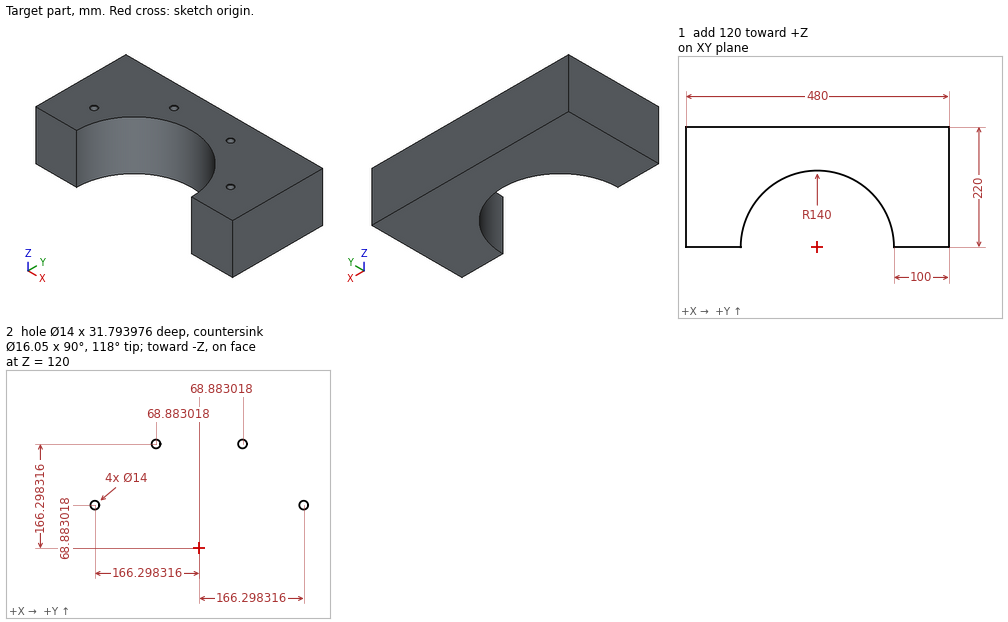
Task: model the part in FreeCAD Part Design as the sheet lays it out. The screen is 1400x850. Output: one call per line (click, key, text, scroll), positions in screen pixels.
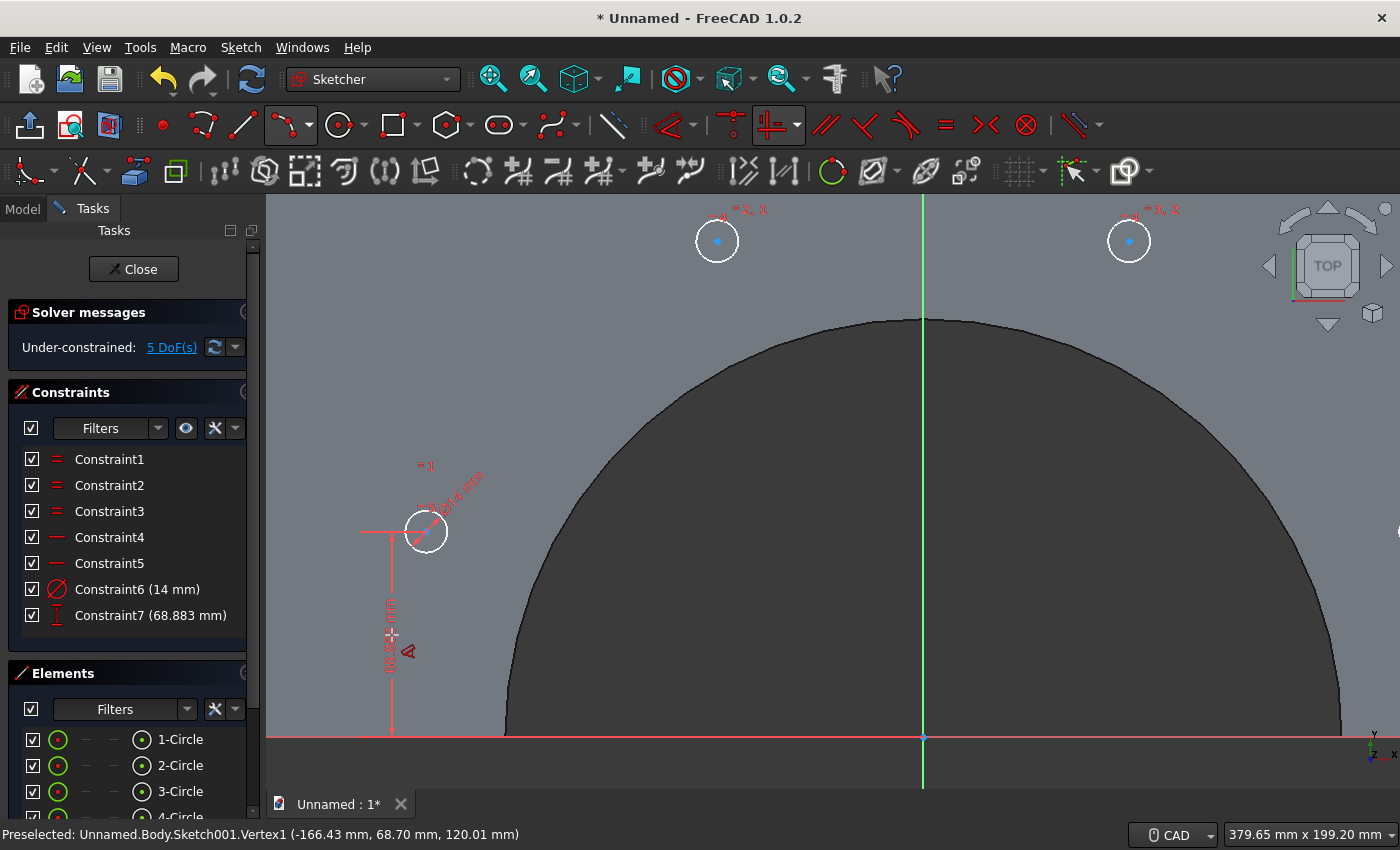
click(717, 241)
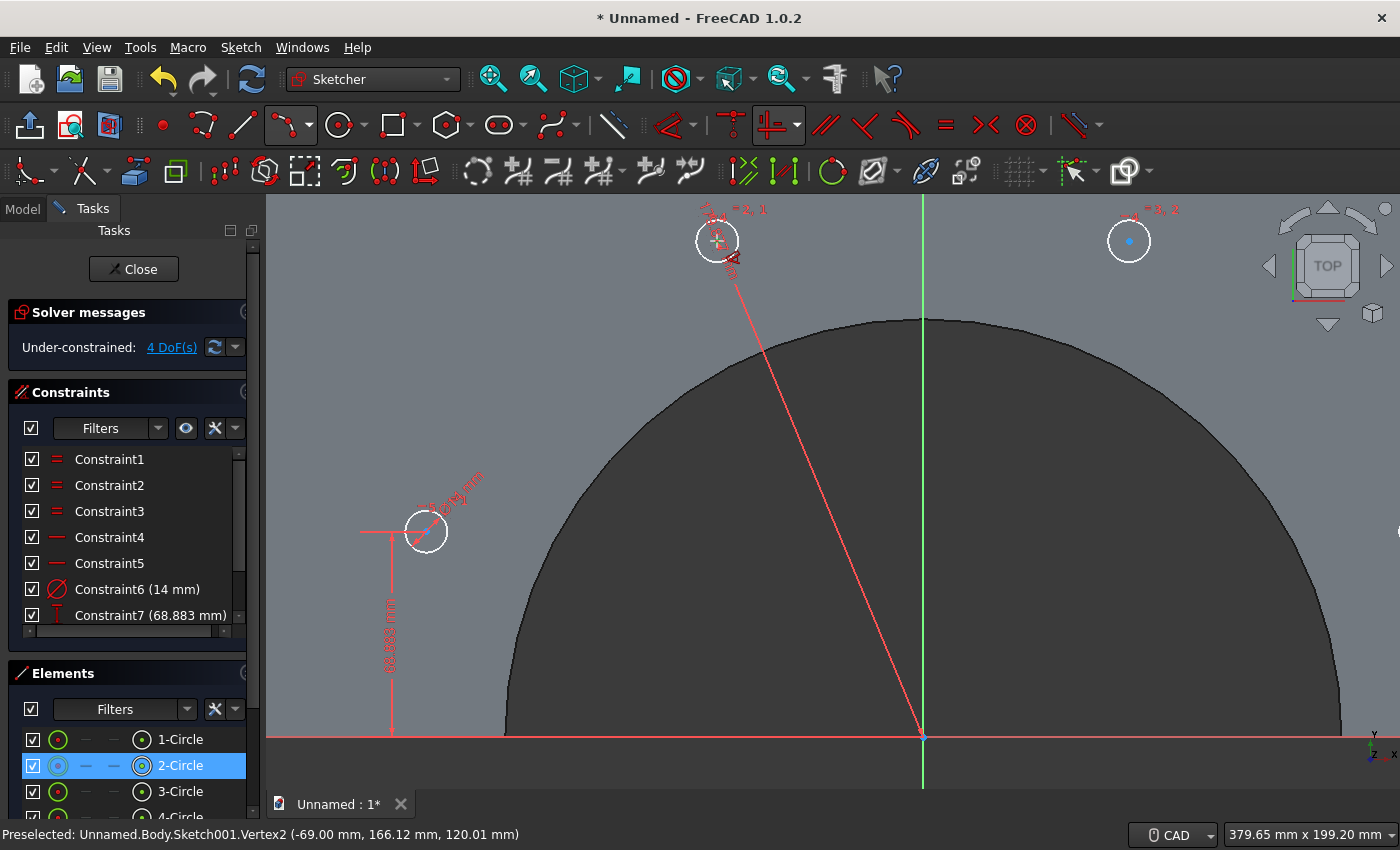
key(Escape)
key(Escape)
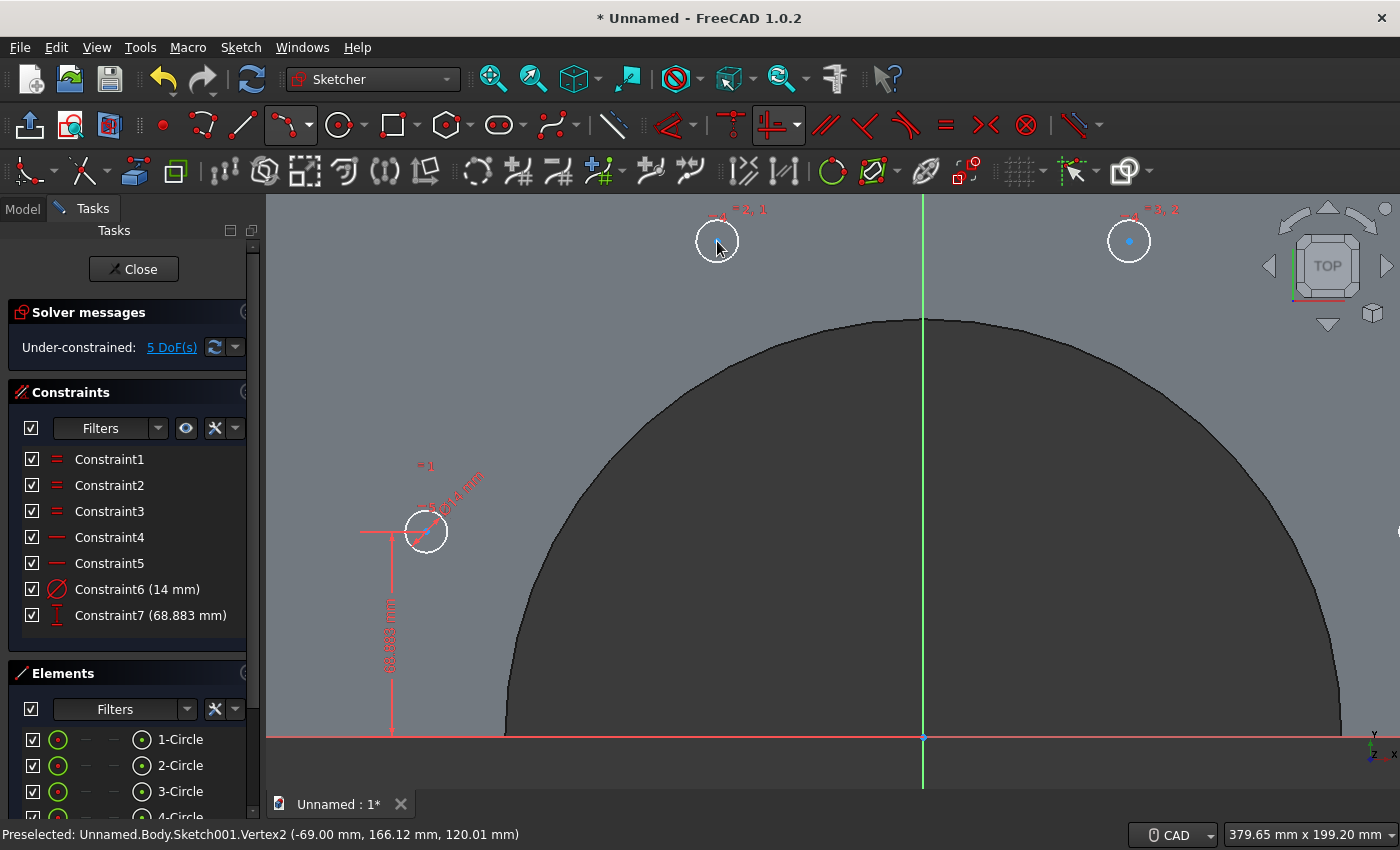
click(717, 241)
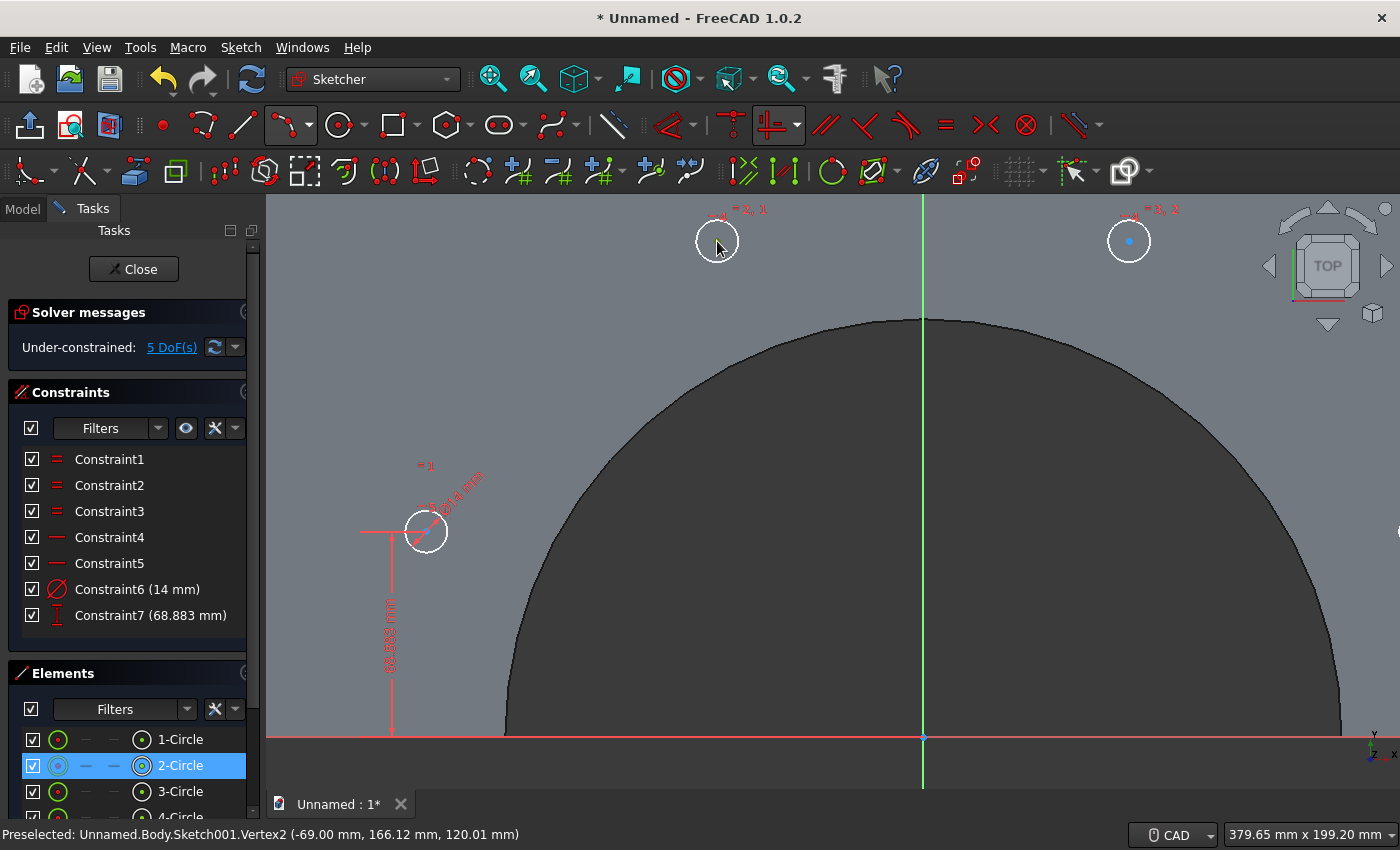
key(l)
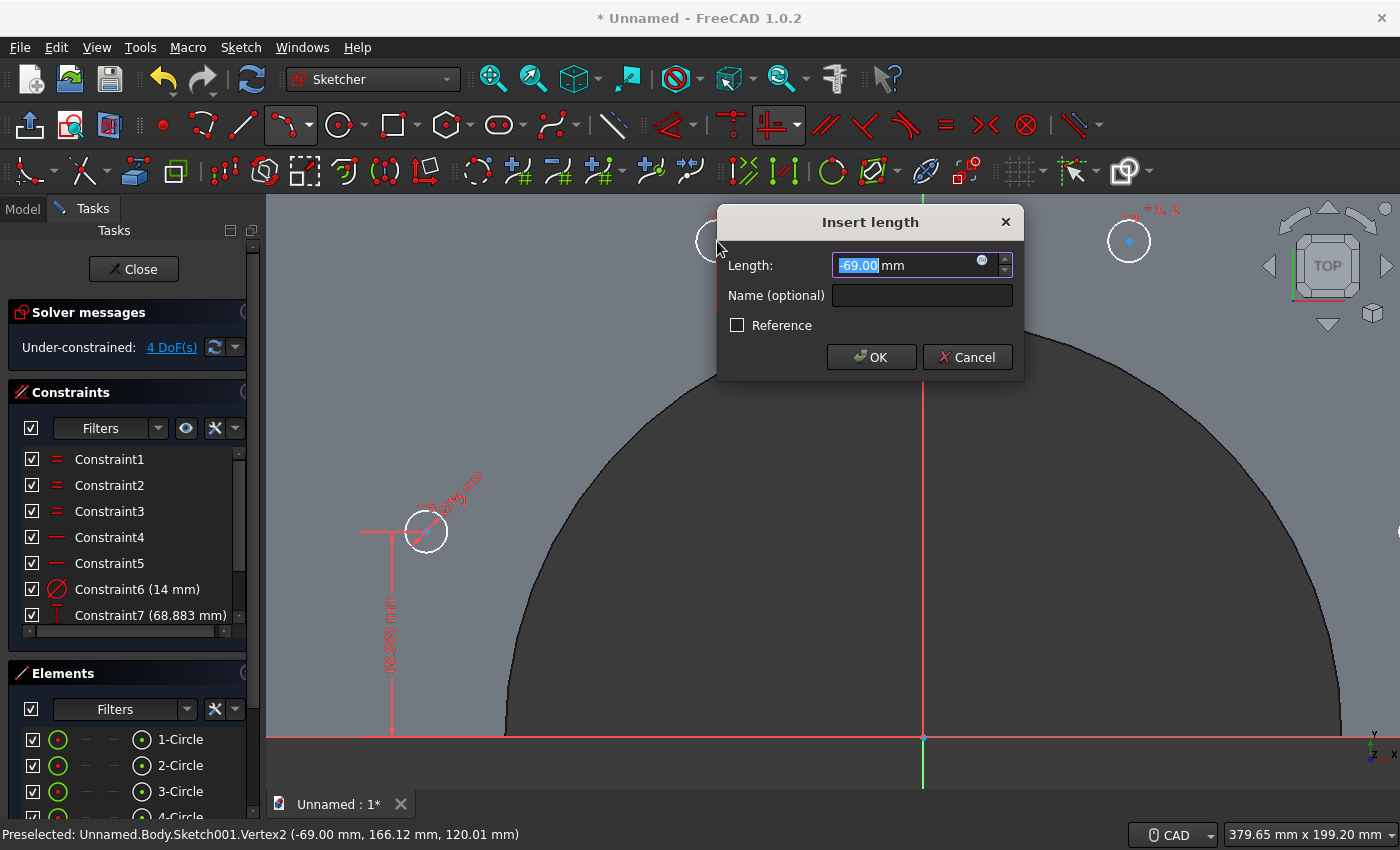
text(-68.883018)
key(Return)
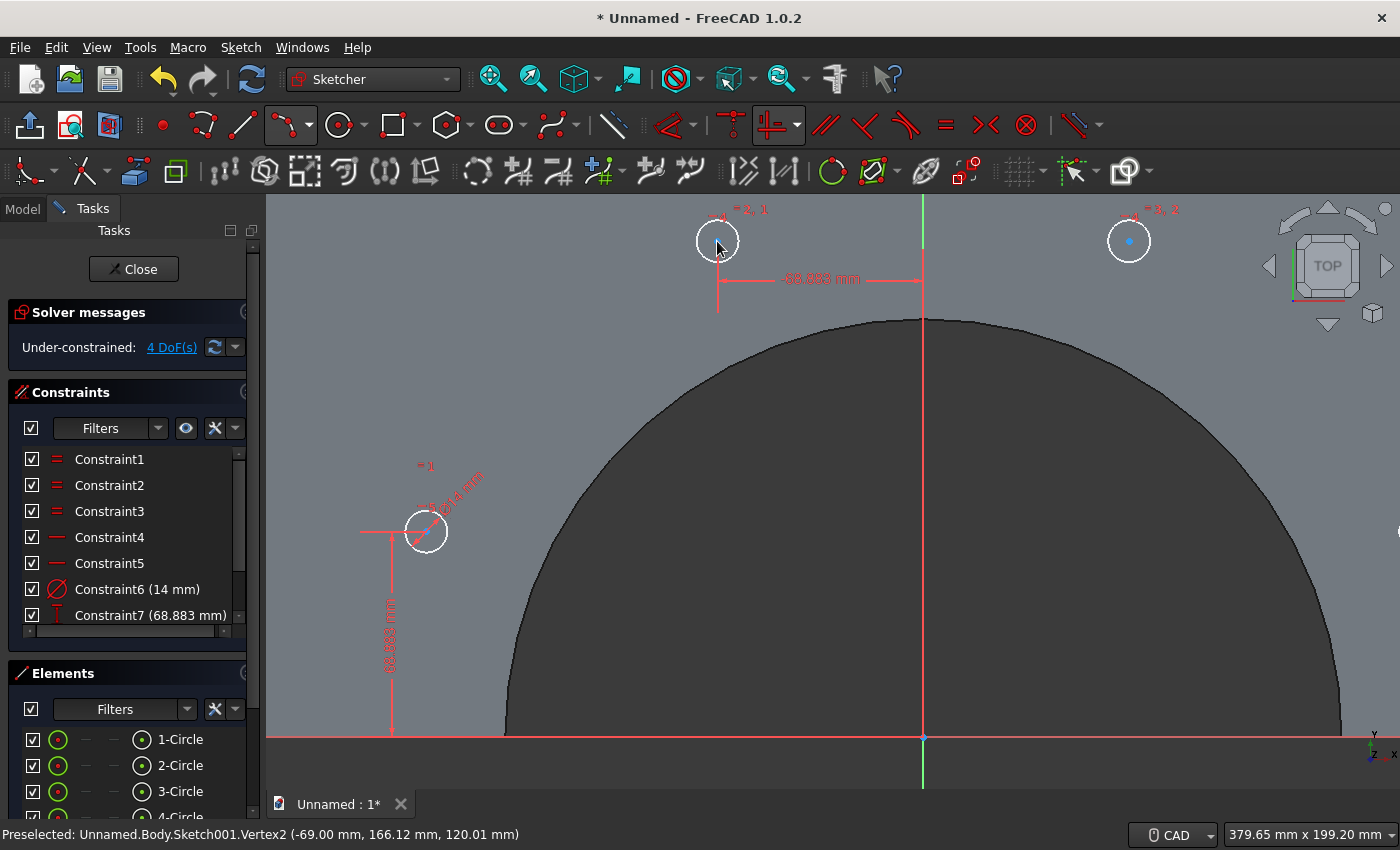
click(1129, 241)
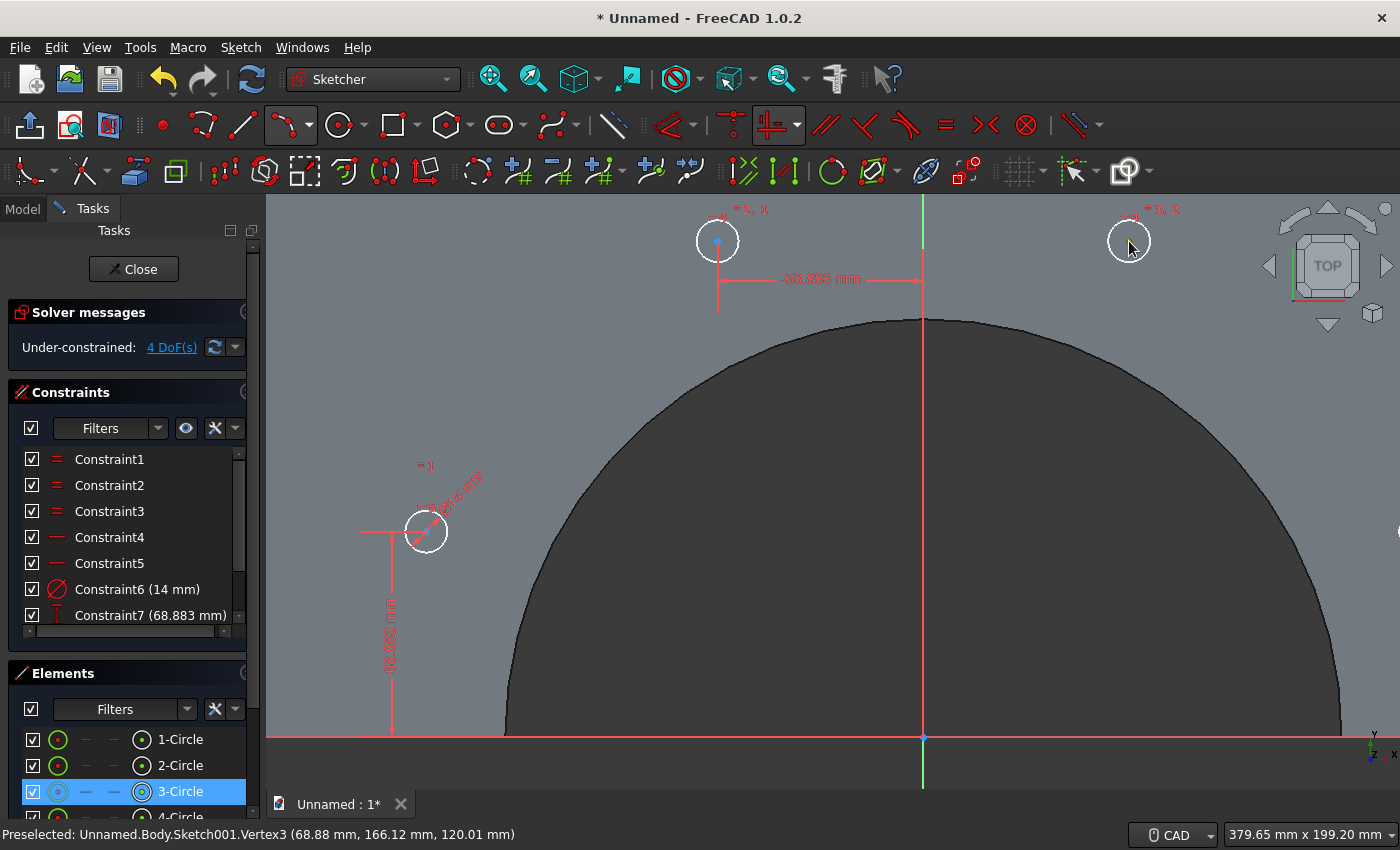
click(696, 126)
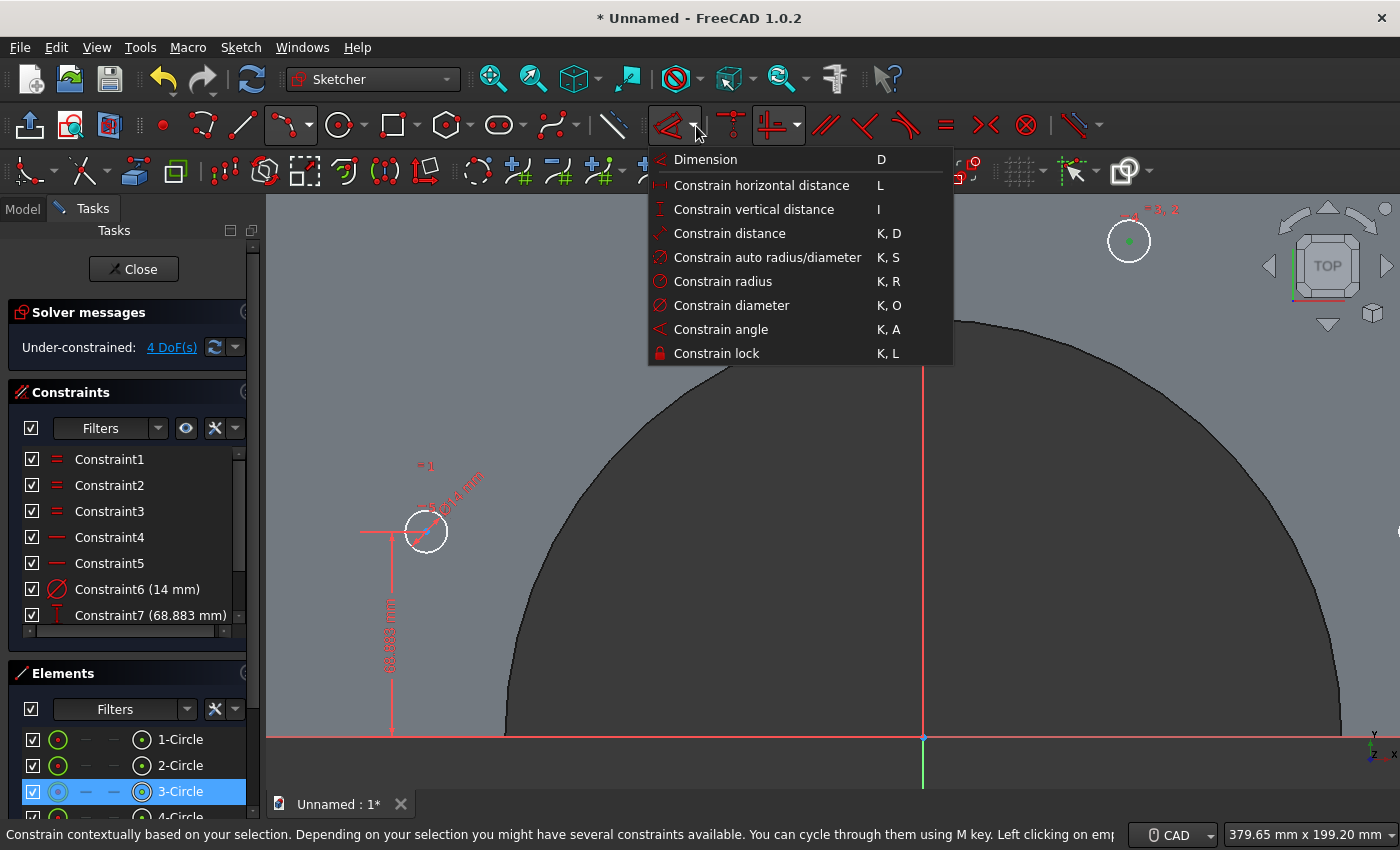
click(801, 185)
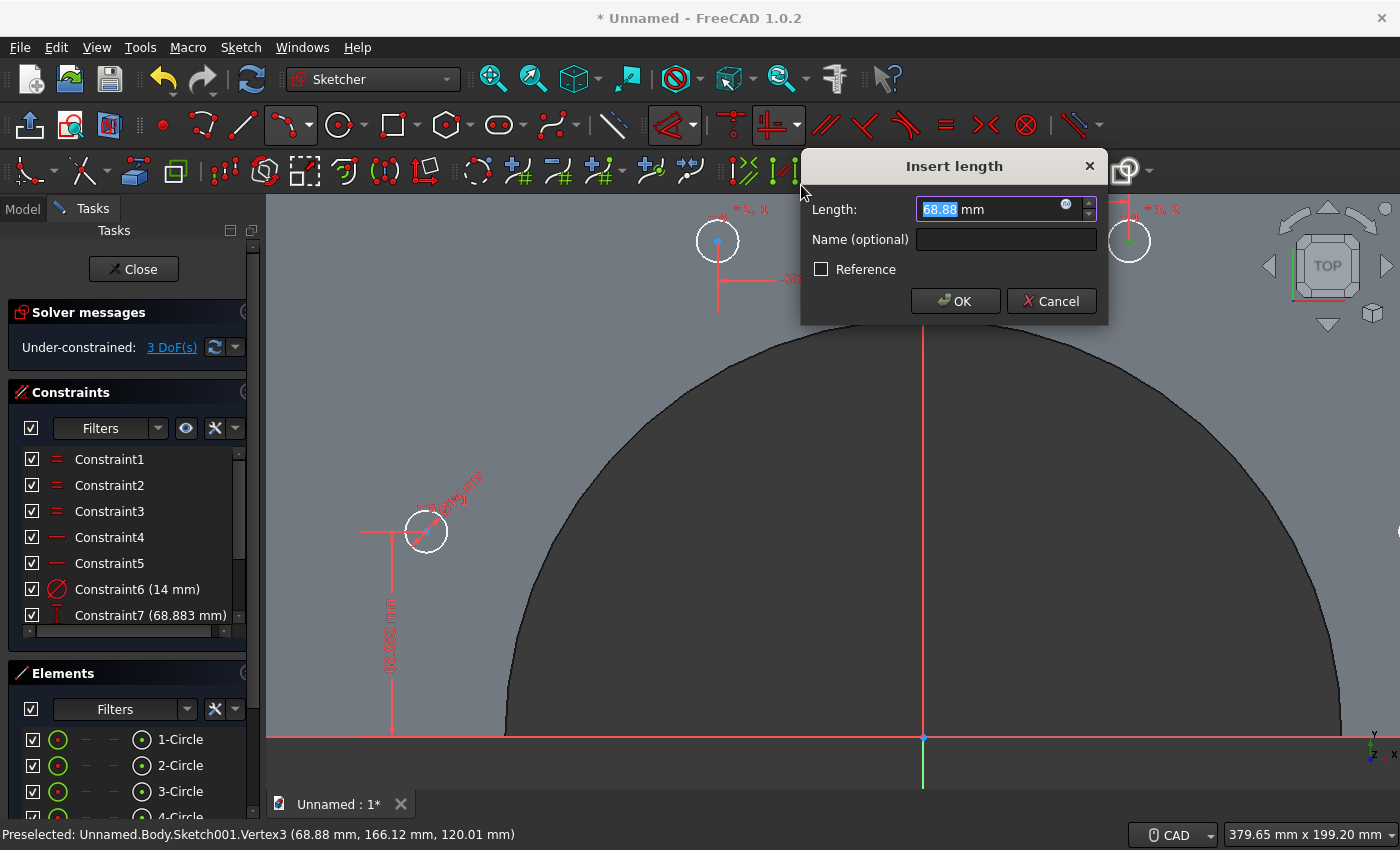
text(68.883018)
key(Return)